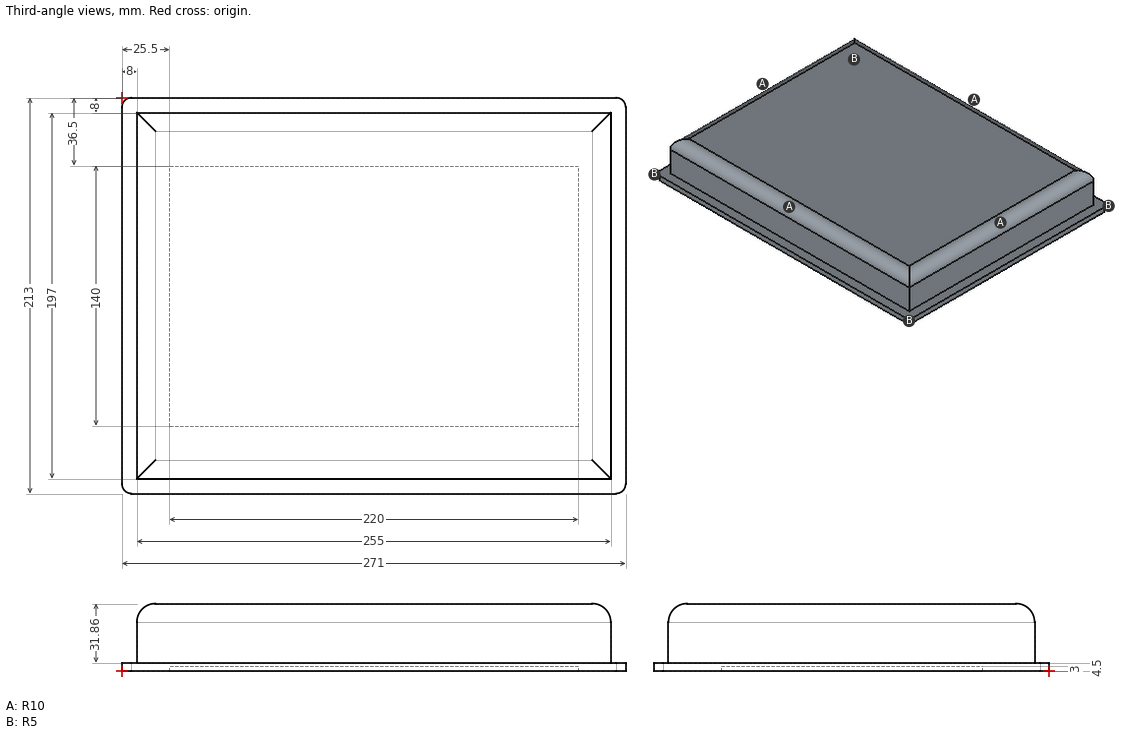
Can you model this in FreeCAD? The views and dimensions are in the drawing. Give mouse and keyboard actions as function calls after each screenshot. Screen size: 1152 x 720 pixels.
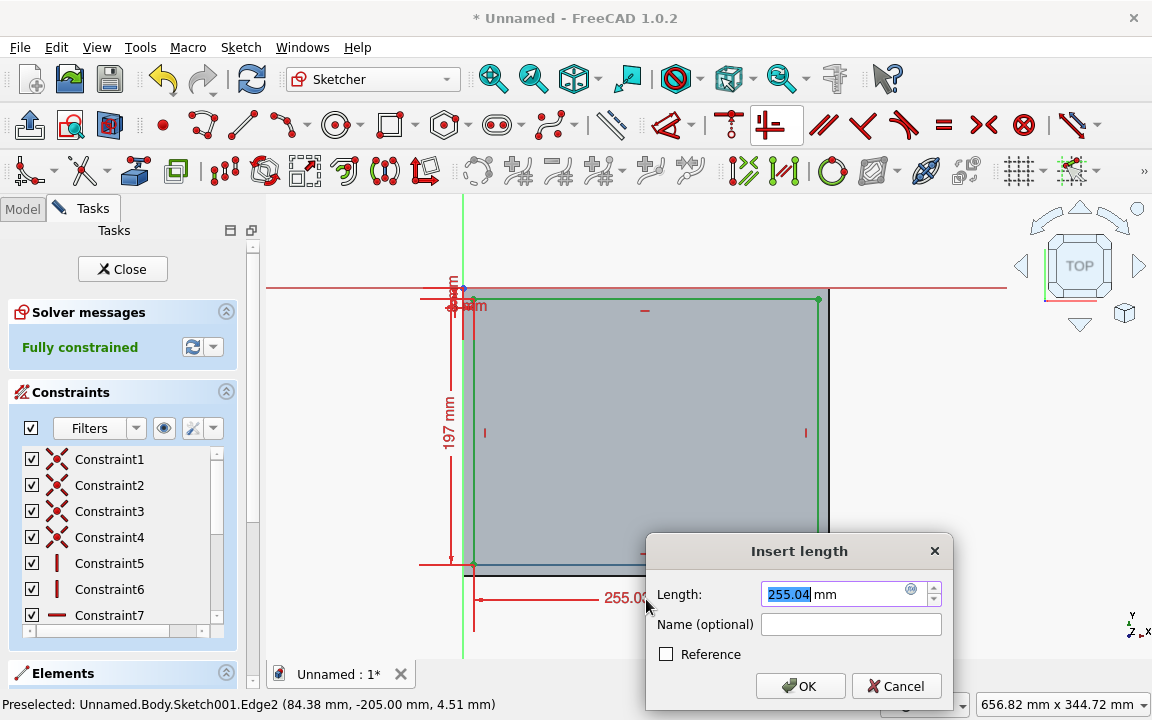
text(255)
key(Return)
key(Escape)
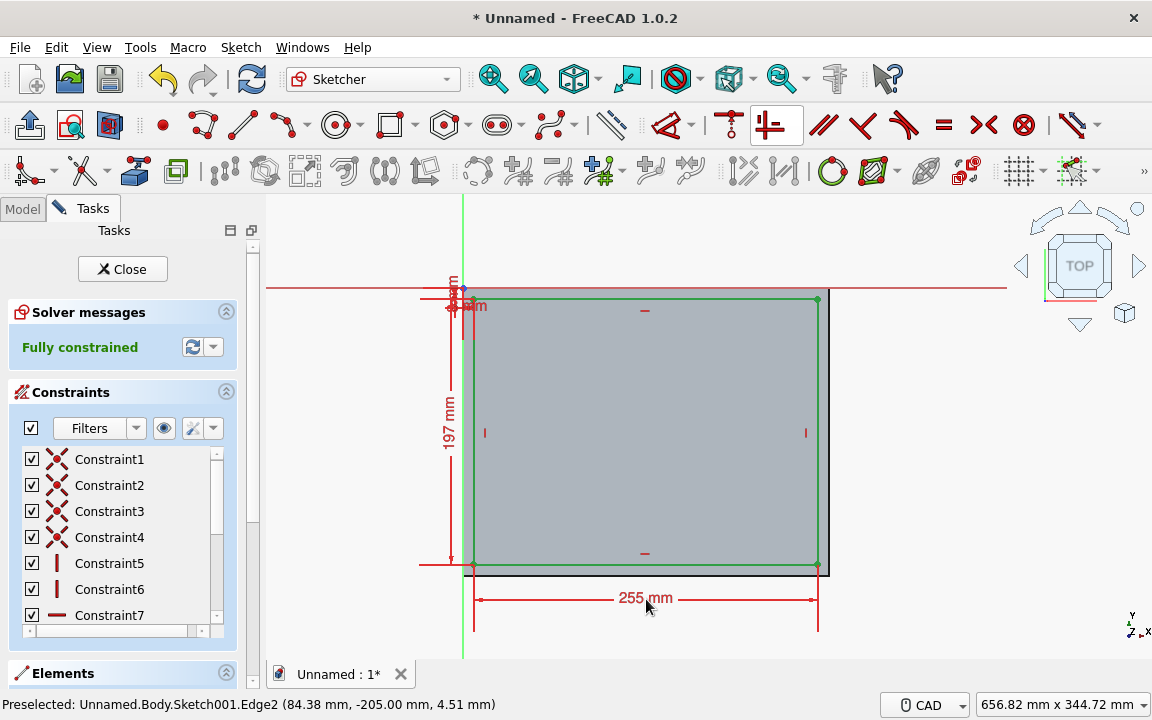
click(123, 269)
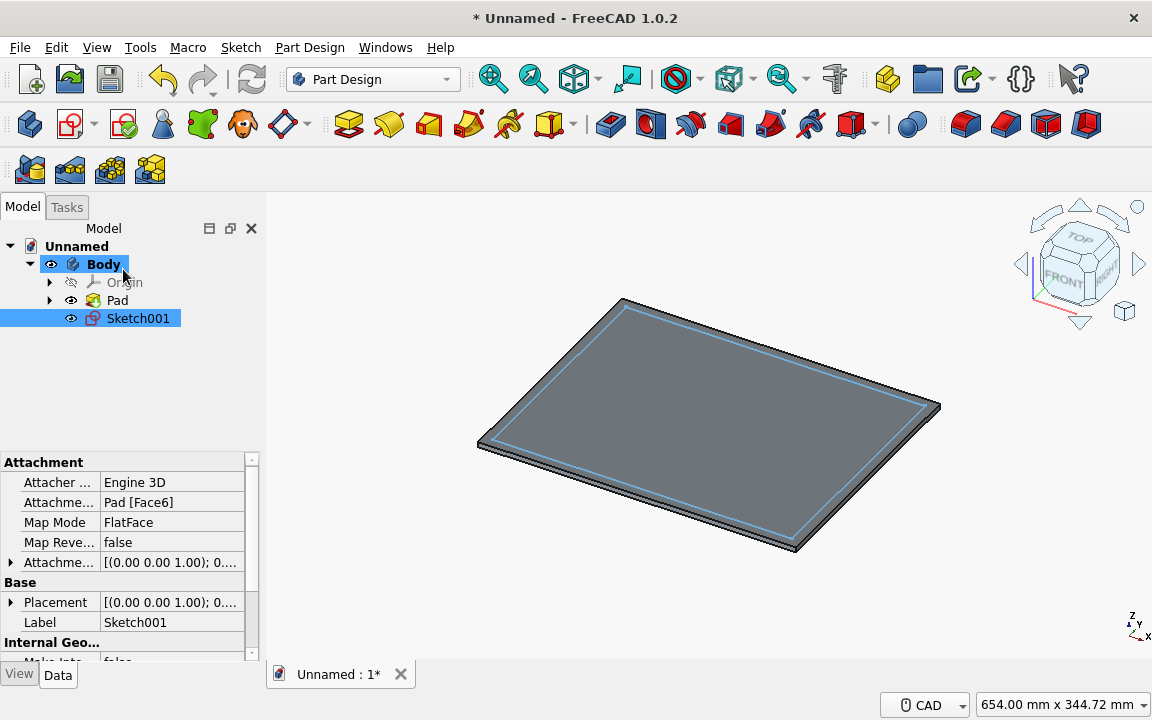
click(350, 124)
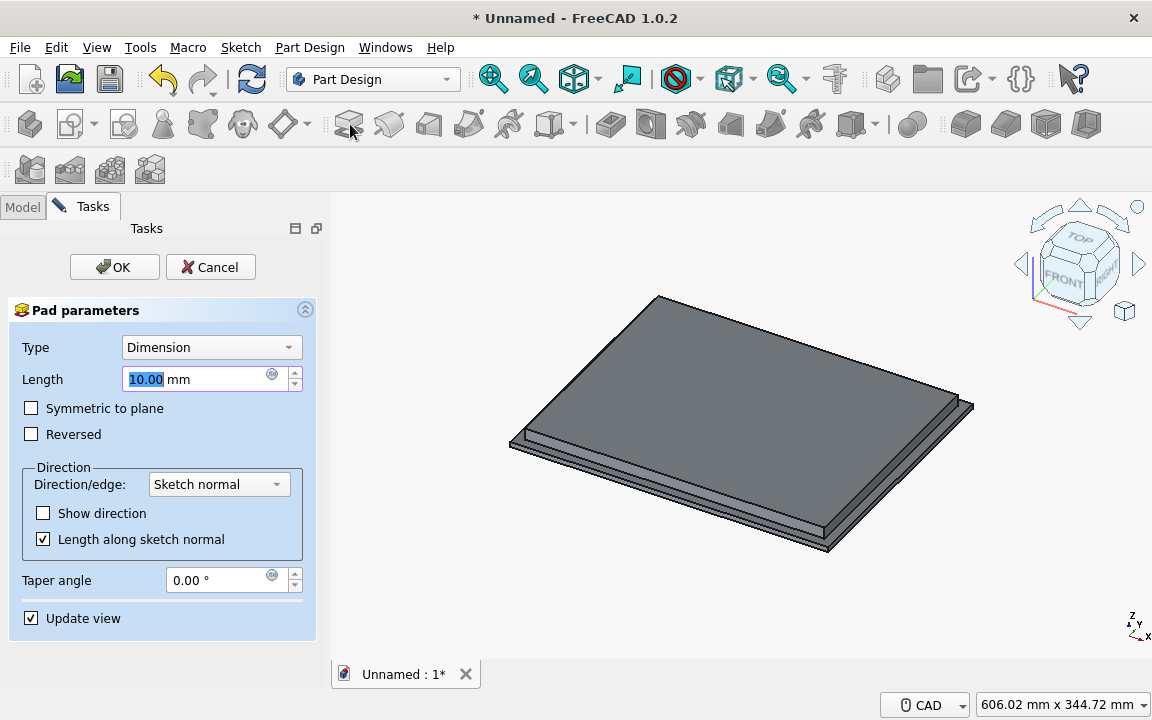
text(31.86)
key(Tab)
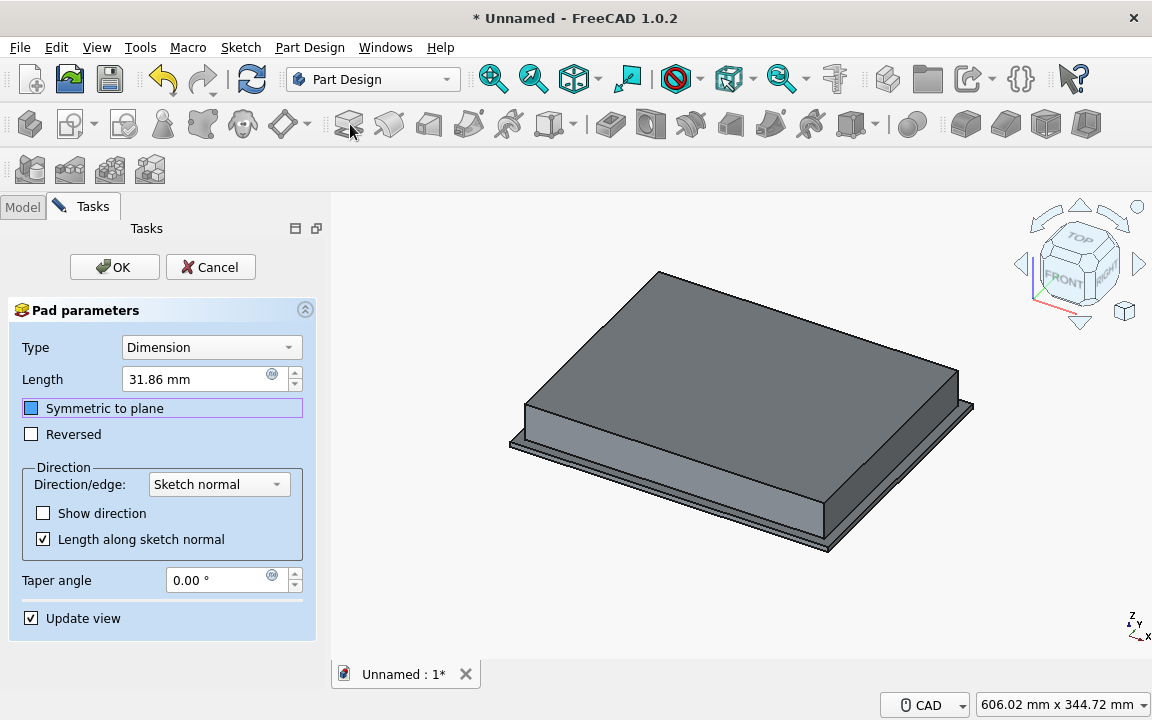
click(115, 267)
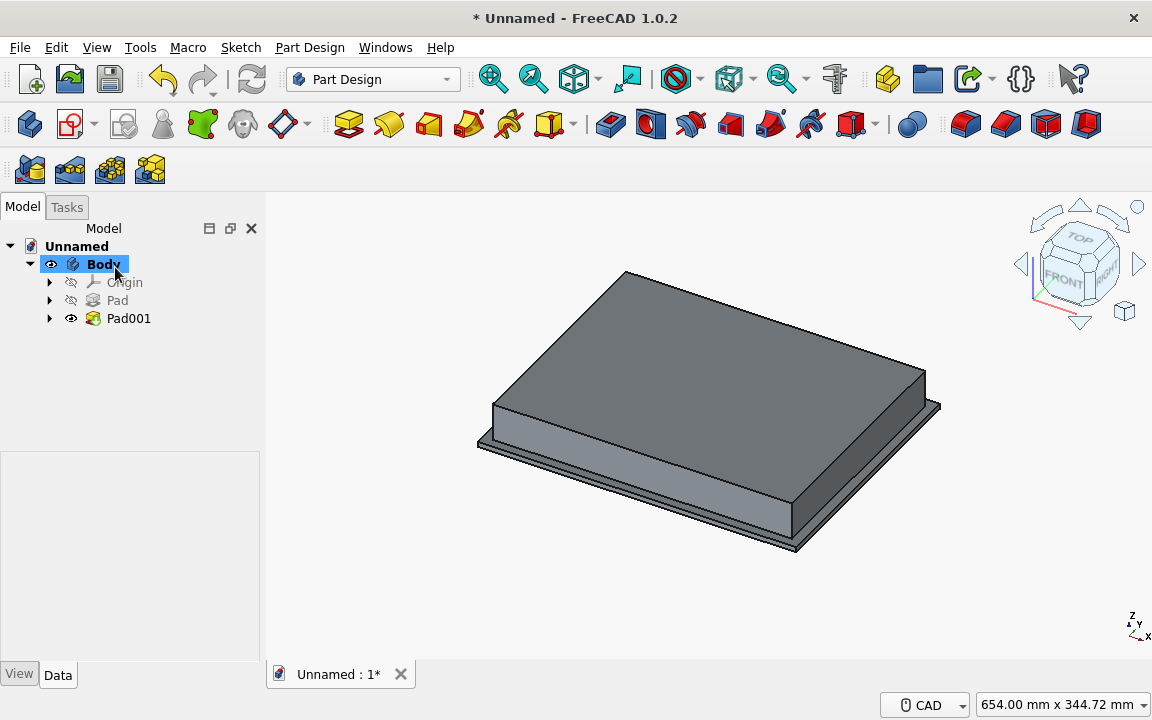
click(709, 387)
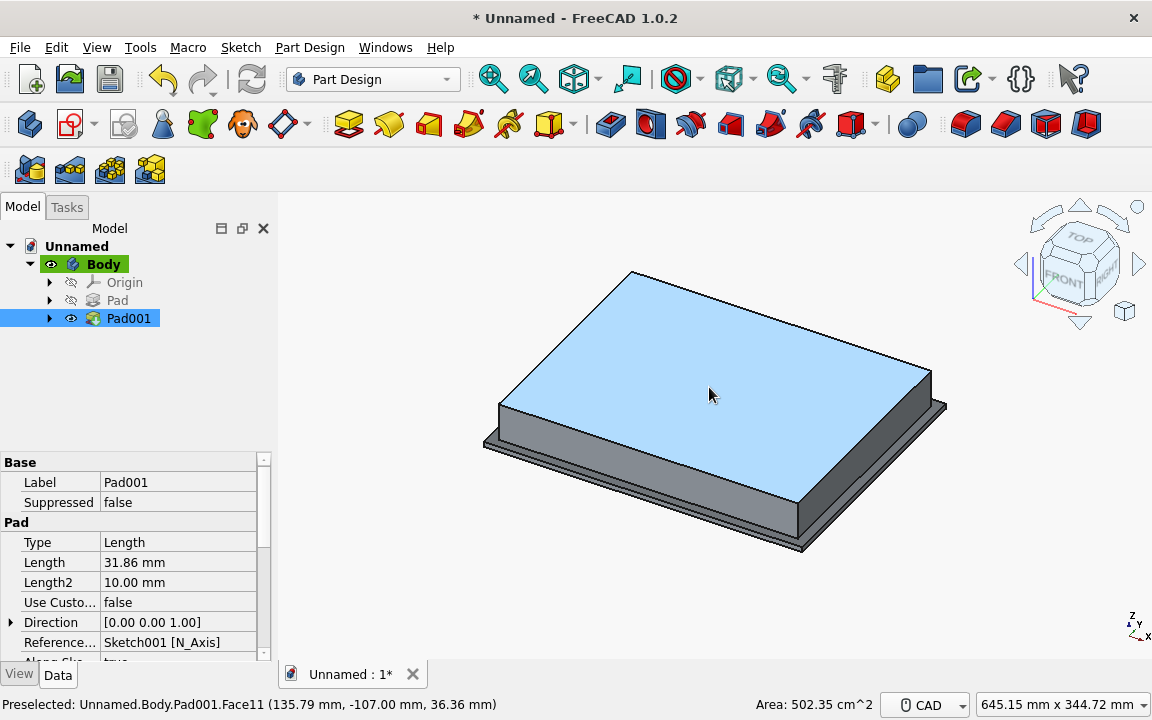
click(966, 124)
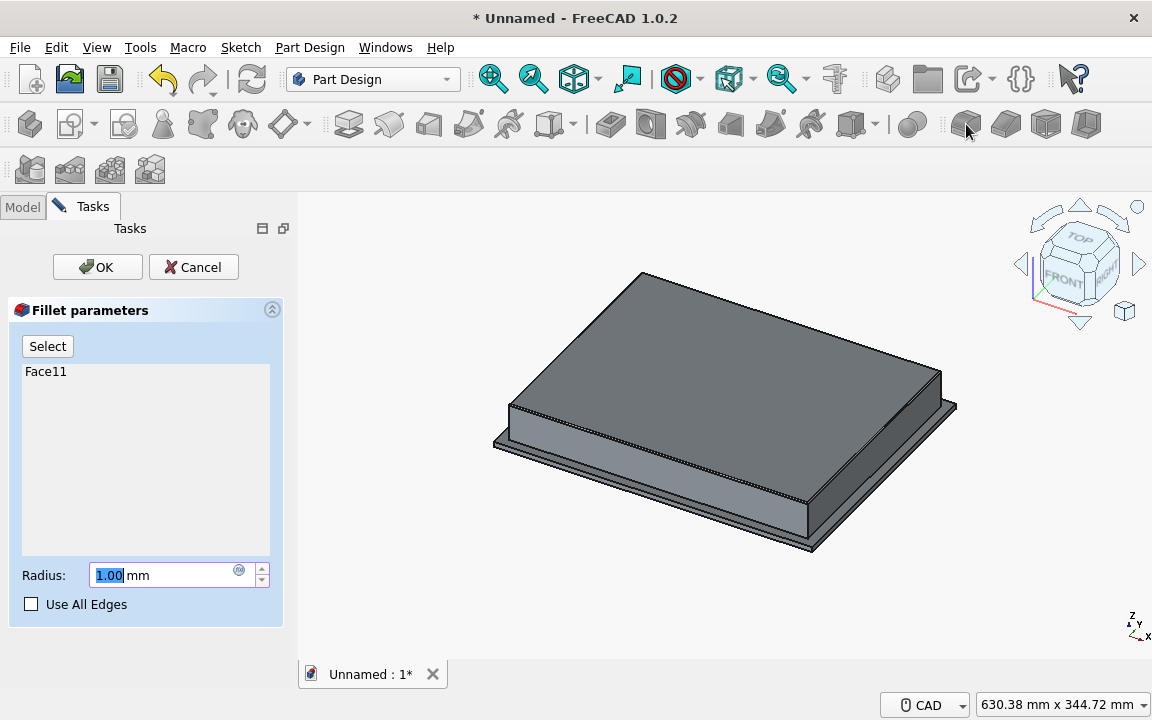
text(10)
key(Tab)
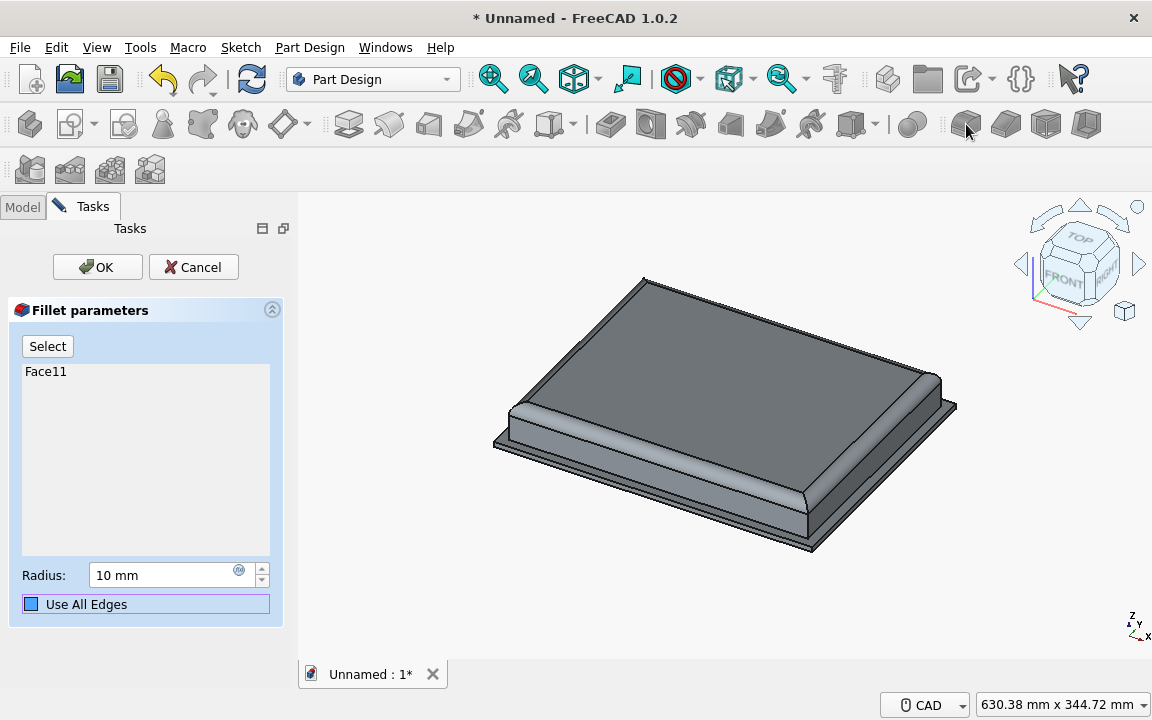
click(98, 267)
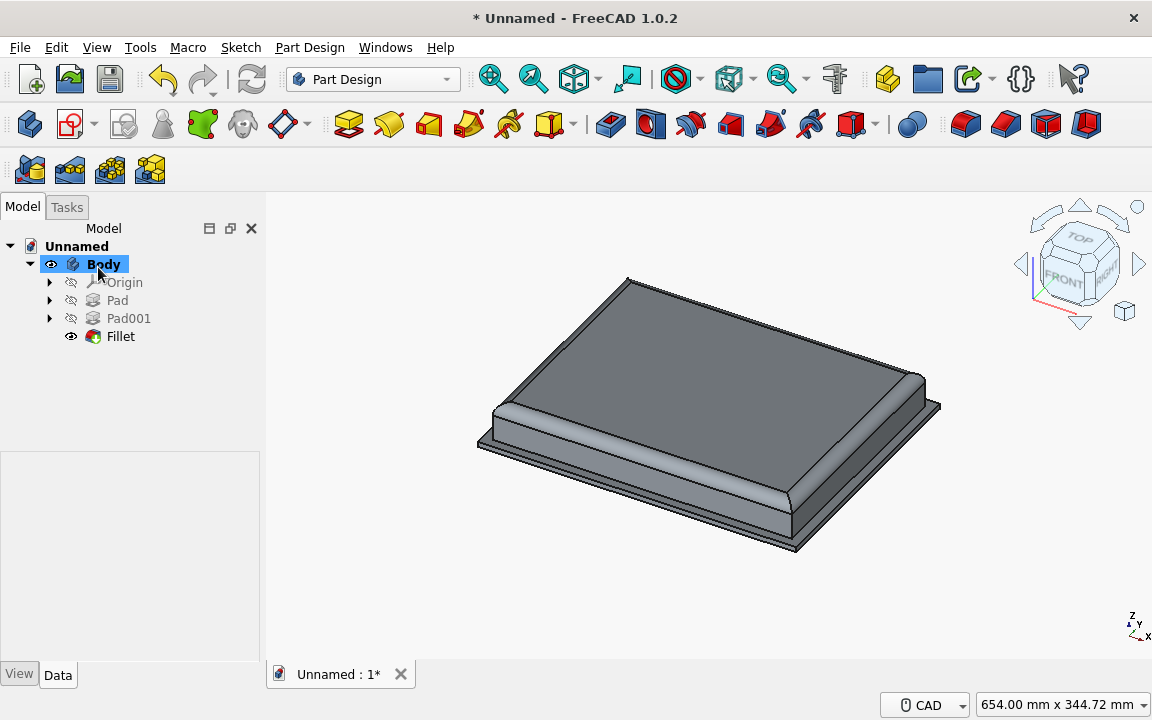
scroll(622, 300, up, 10)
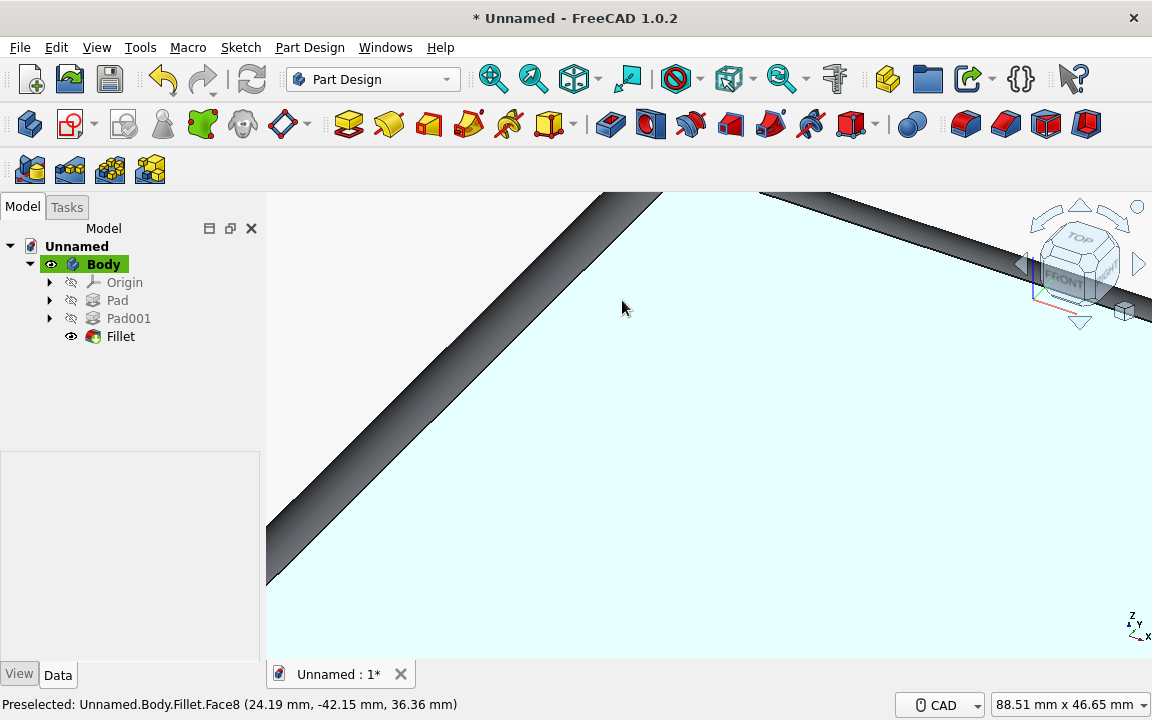
click(494, 80)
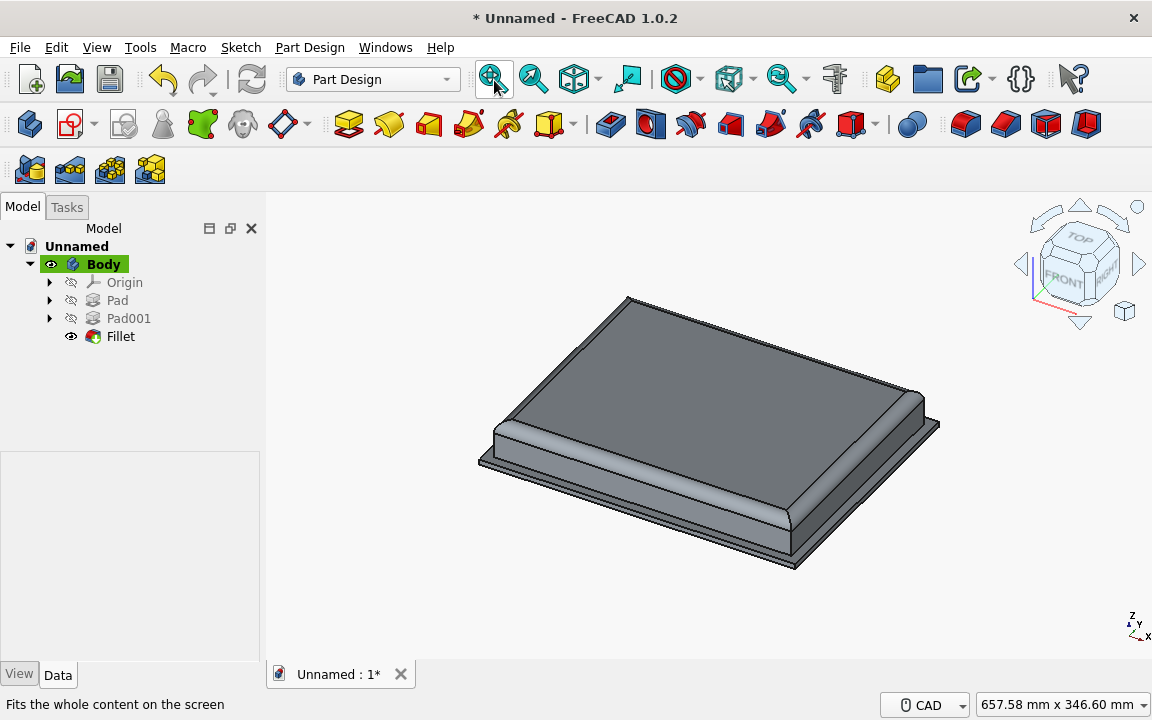
key(0)